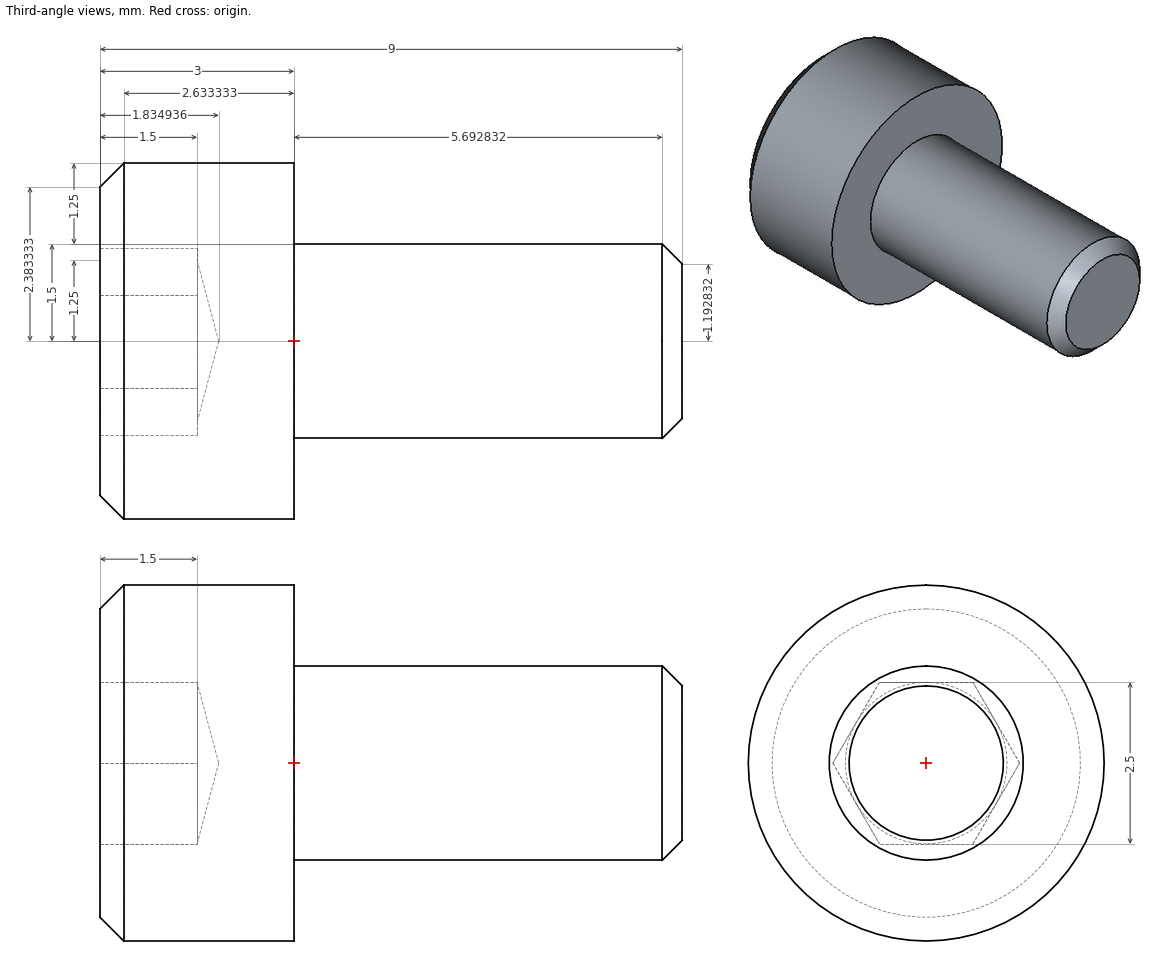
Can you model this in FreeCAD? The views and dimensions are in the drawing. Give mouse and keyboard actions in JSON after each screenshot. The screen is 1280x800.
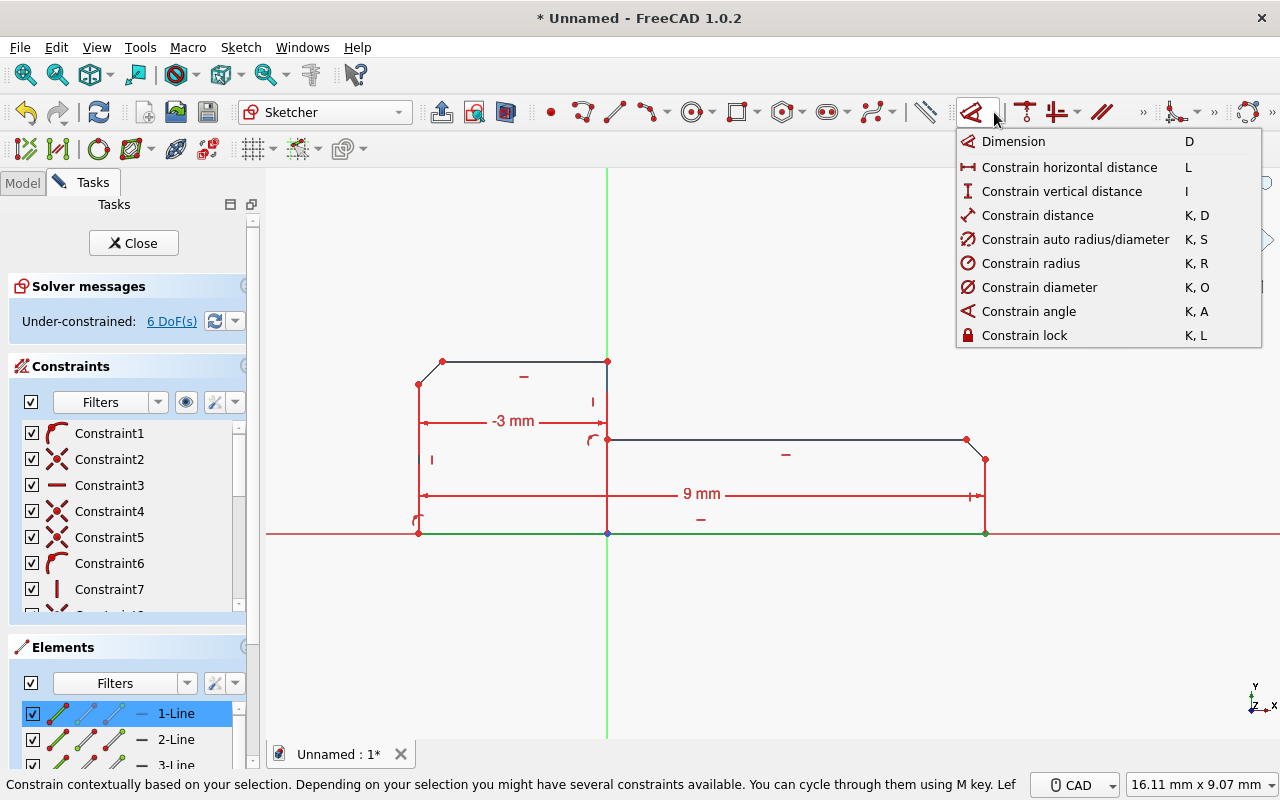
{"action": "left_click", "coordinate": [1109, 191]}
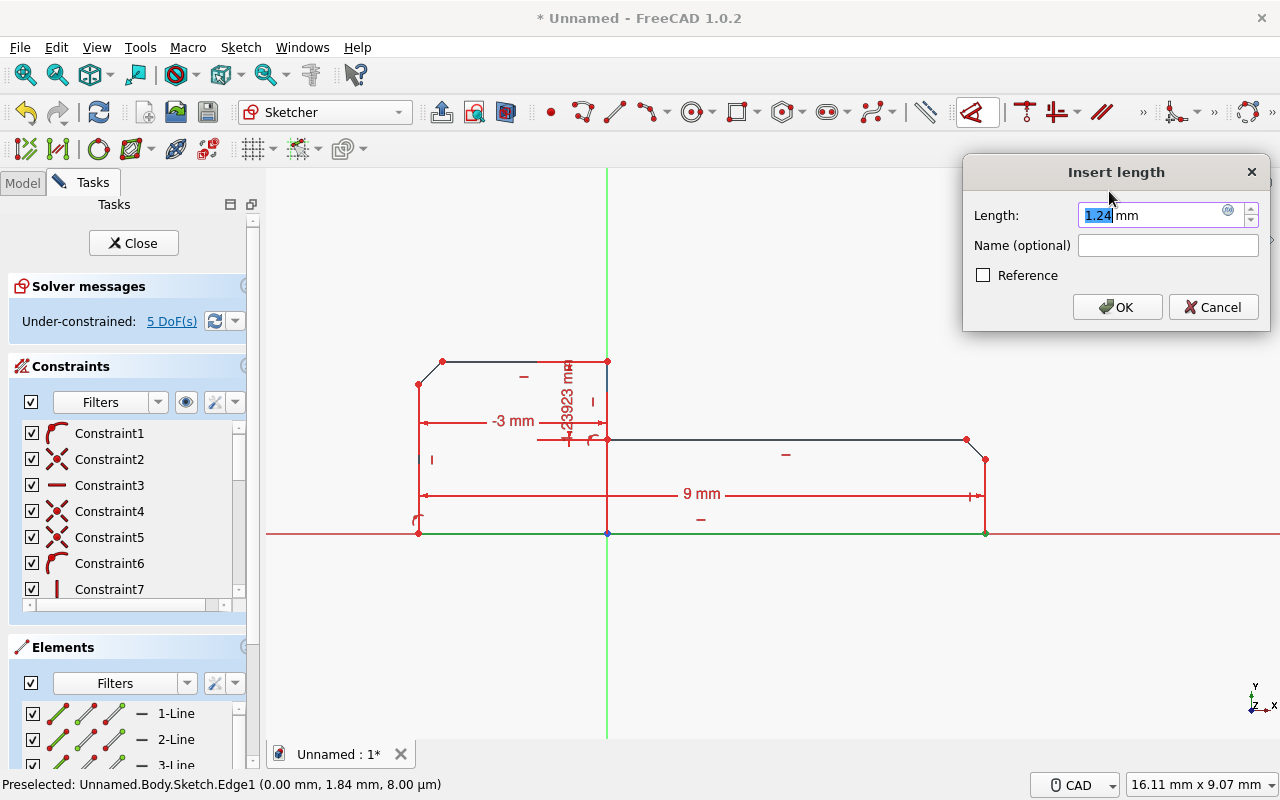
{"action": "type", "text": "1.25"}
{"action": "key", "text": "Return"}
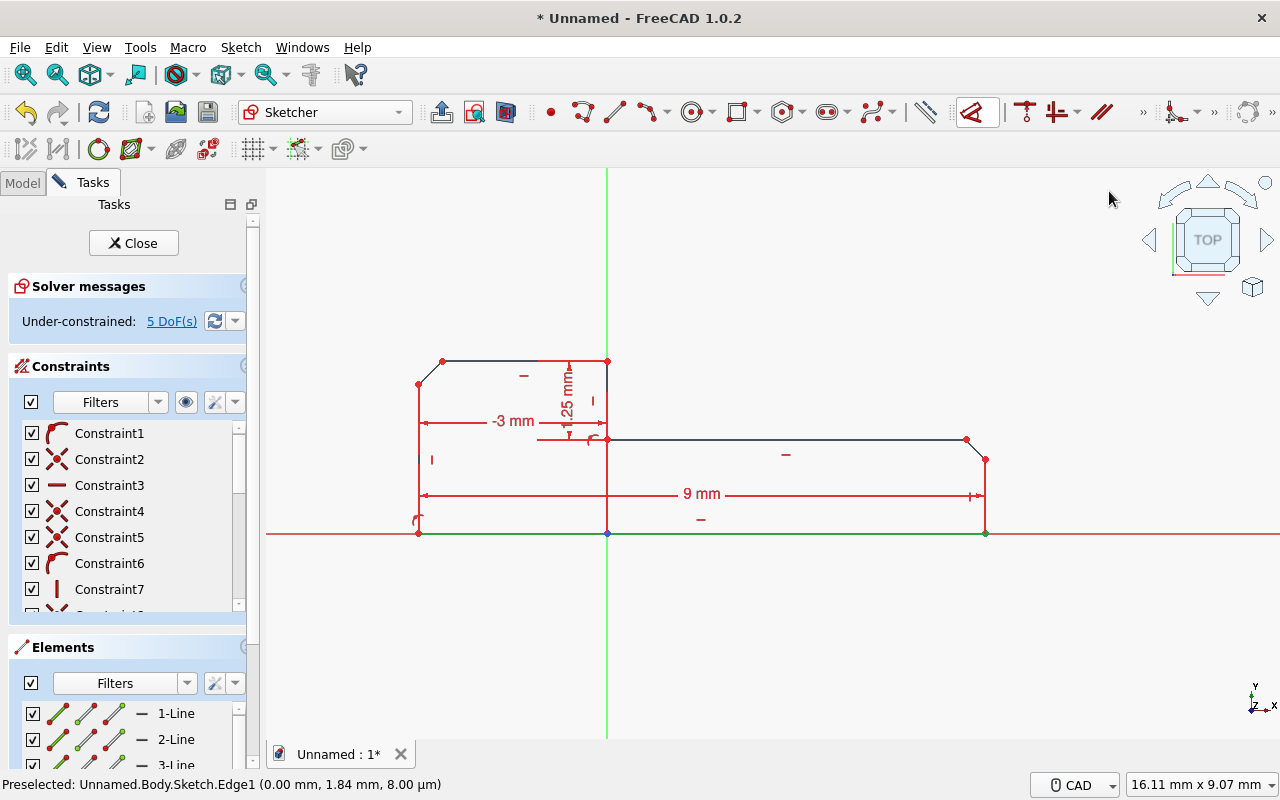
{"action": "left_click", "coordinate": [607, 440]}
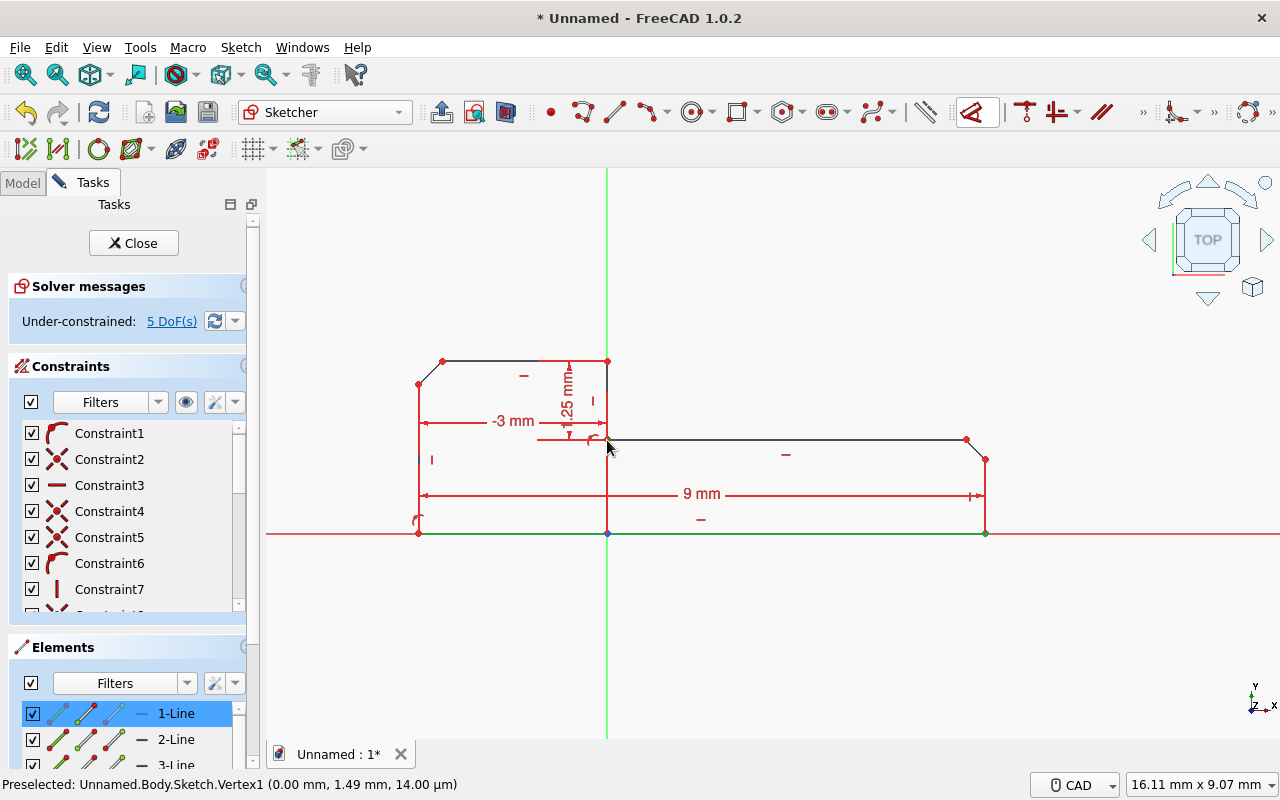
{"action": "left_click", "coordinate": [994, 112]}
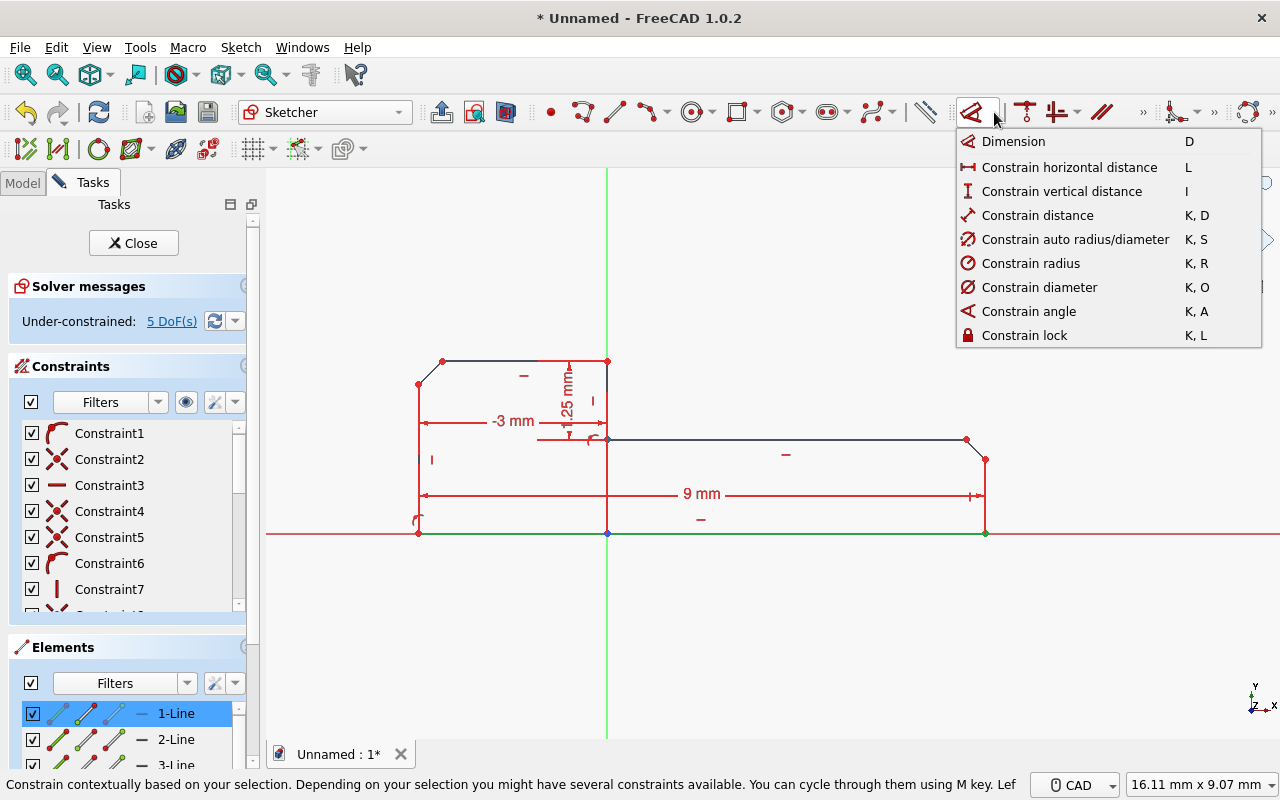
{"action": "left_click", "coordinate": [1109, 191]}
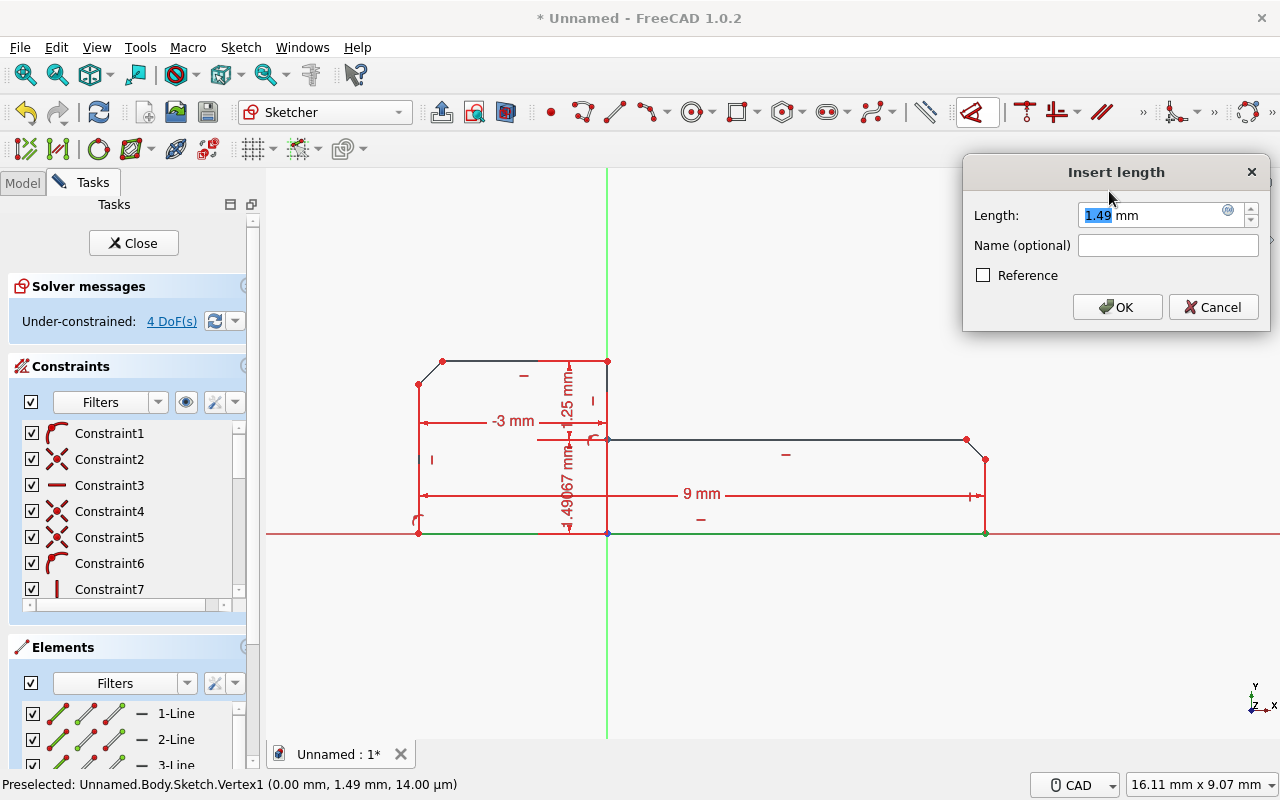
{"action": "type", "text": "1.5"}
{"action": "key", "text": "Return"}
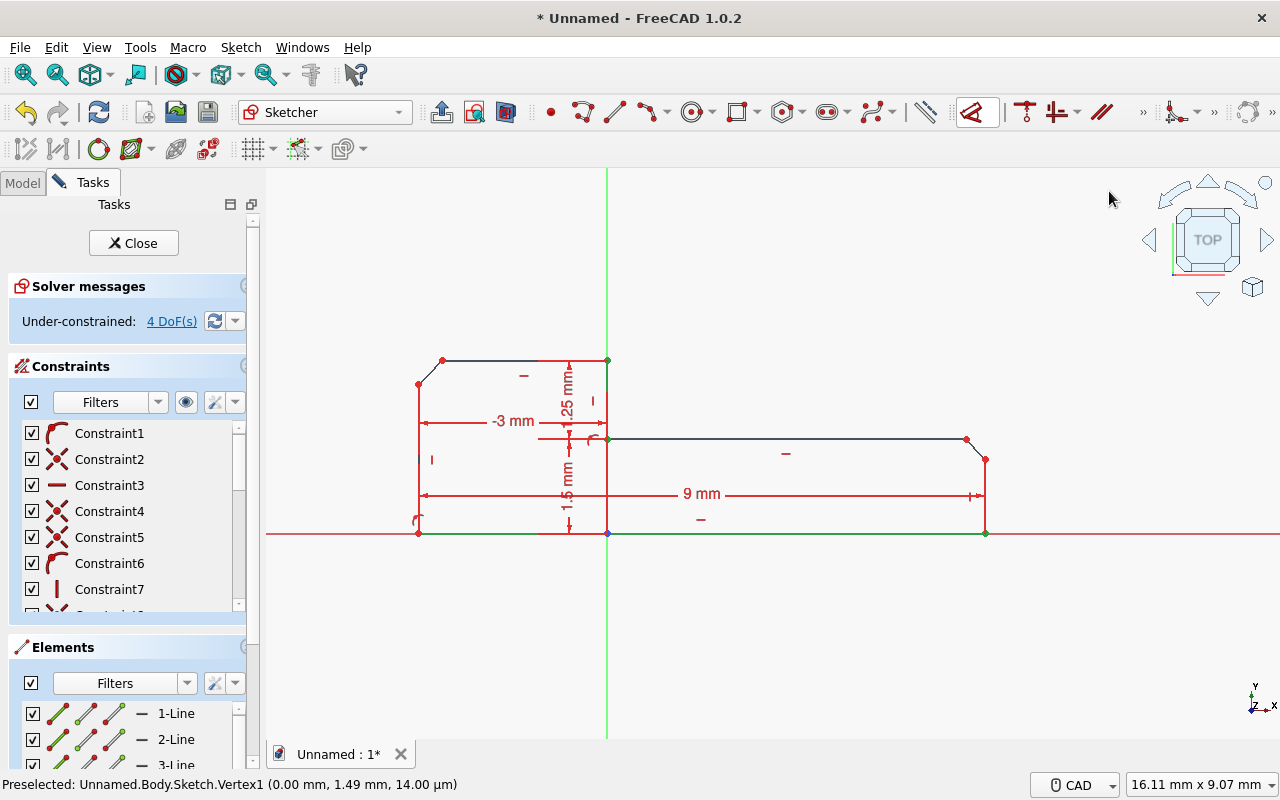
{"action": "left_click", "coordinate": [558, 361]}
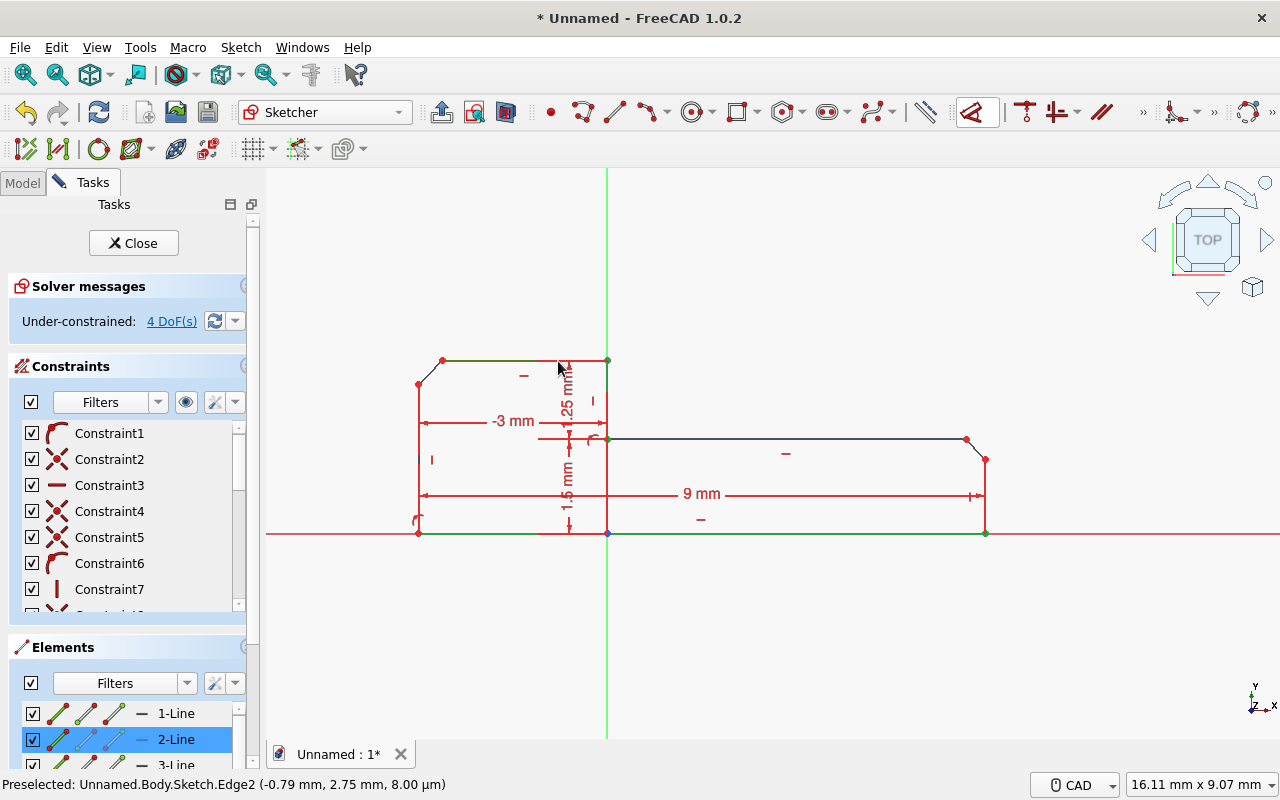
{"action": "left_click", "coordinate": [994, 112]}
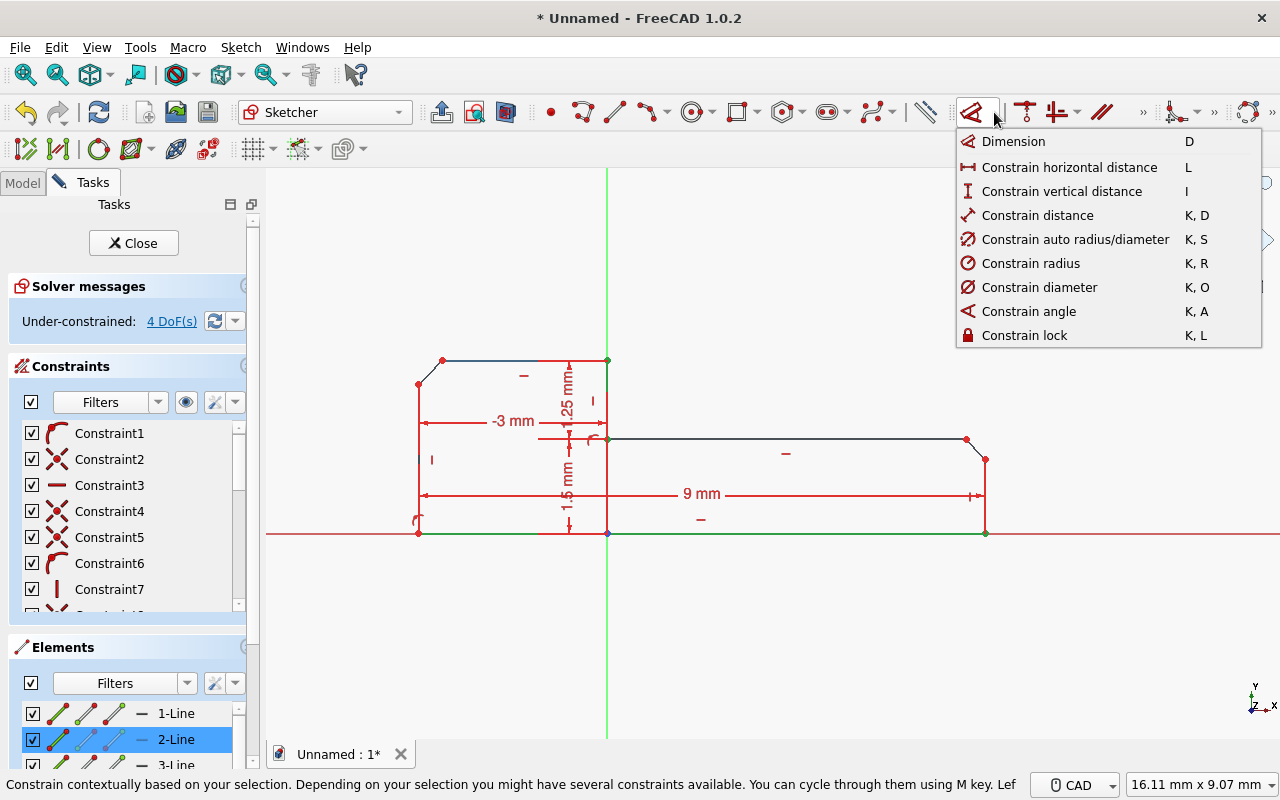
{"action": "left_click", "coordinate": [1109, 167]}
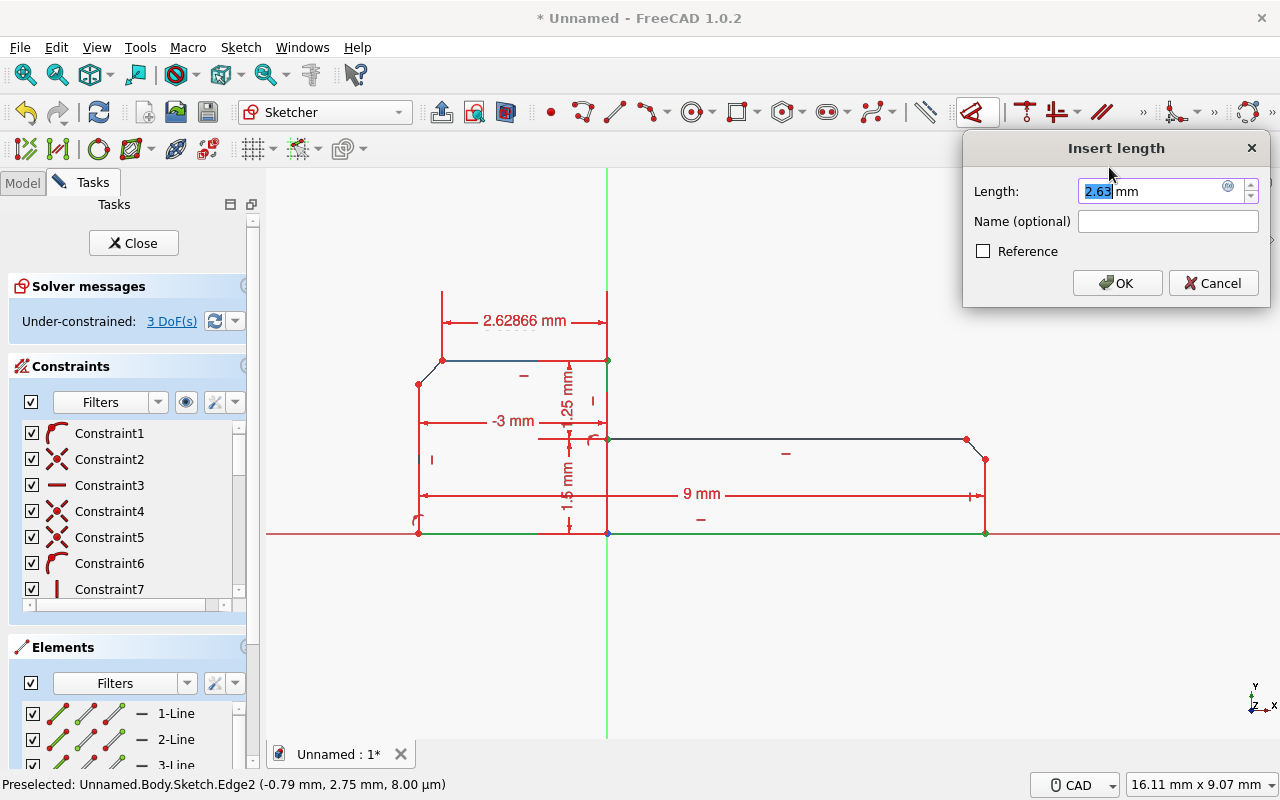
{"action": "type", "text": "2.633333"}
{"action": "key", "text": "Return"}